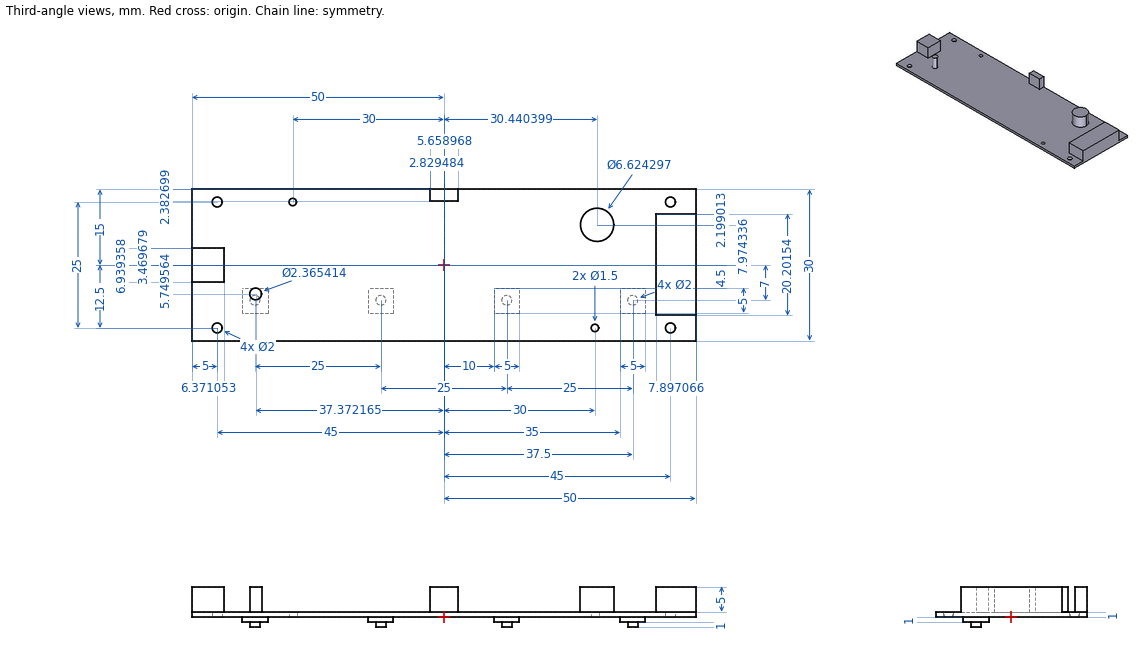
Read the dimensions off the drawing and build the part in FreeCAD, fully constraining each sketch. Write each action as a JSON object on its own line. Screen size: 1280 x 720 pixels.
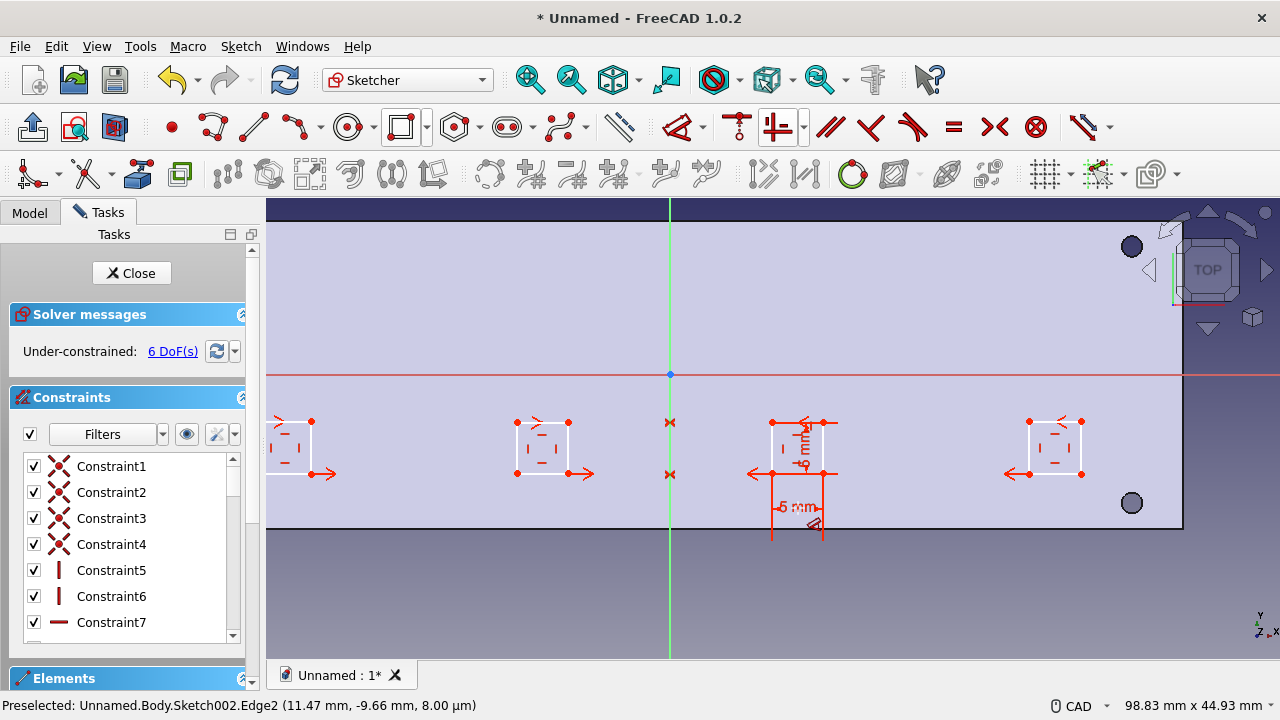
{"action": "left_click", "coordinate": [1029, 437]}
{"action": "left_click", "coordinate": [1063, 448]}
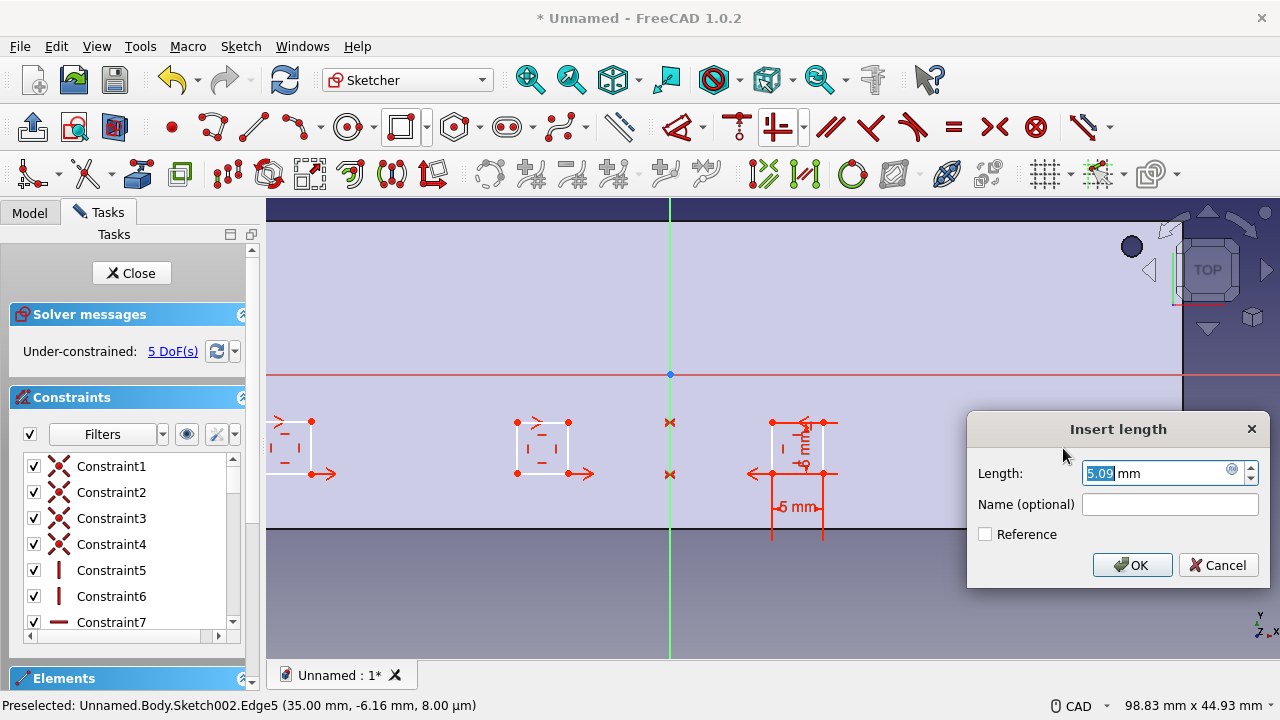
{"action": "type", "text": "5"}
{"action": "key", "text": "Return"}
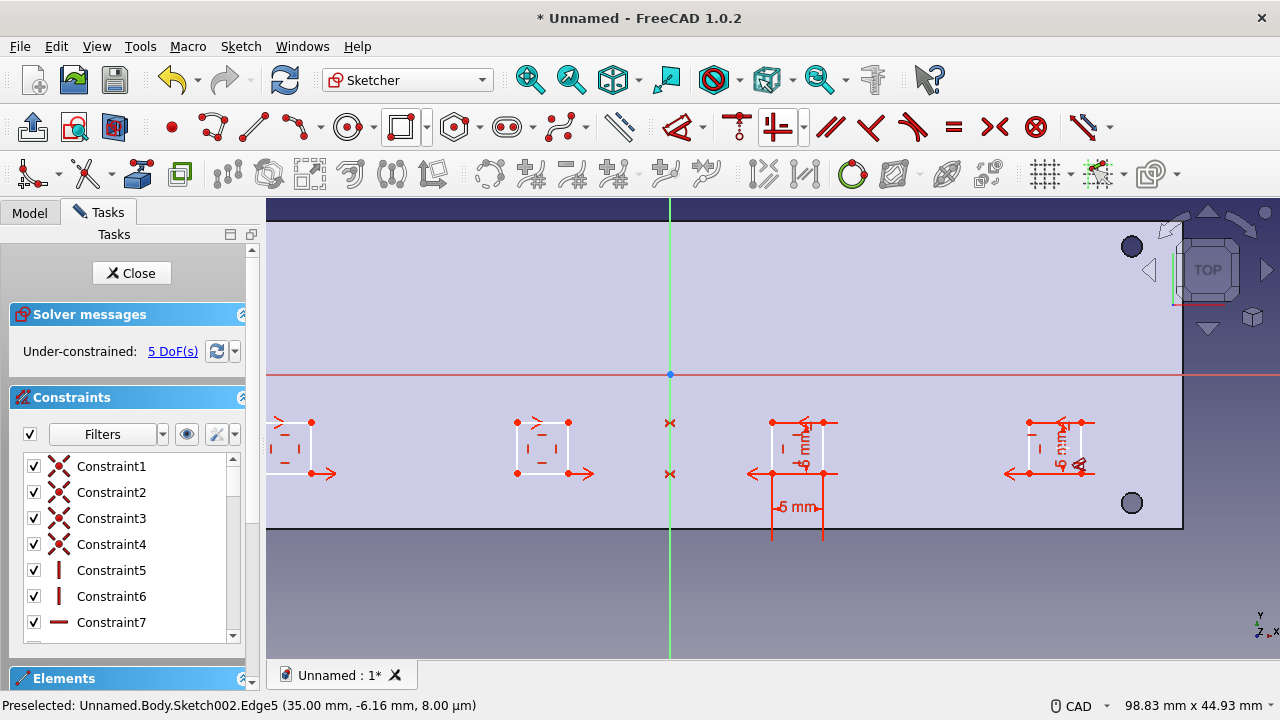
{"action": "left_click", "coordinate": [1045, 474]}
{"action": "left_click", "coordinate": [1055, 508]}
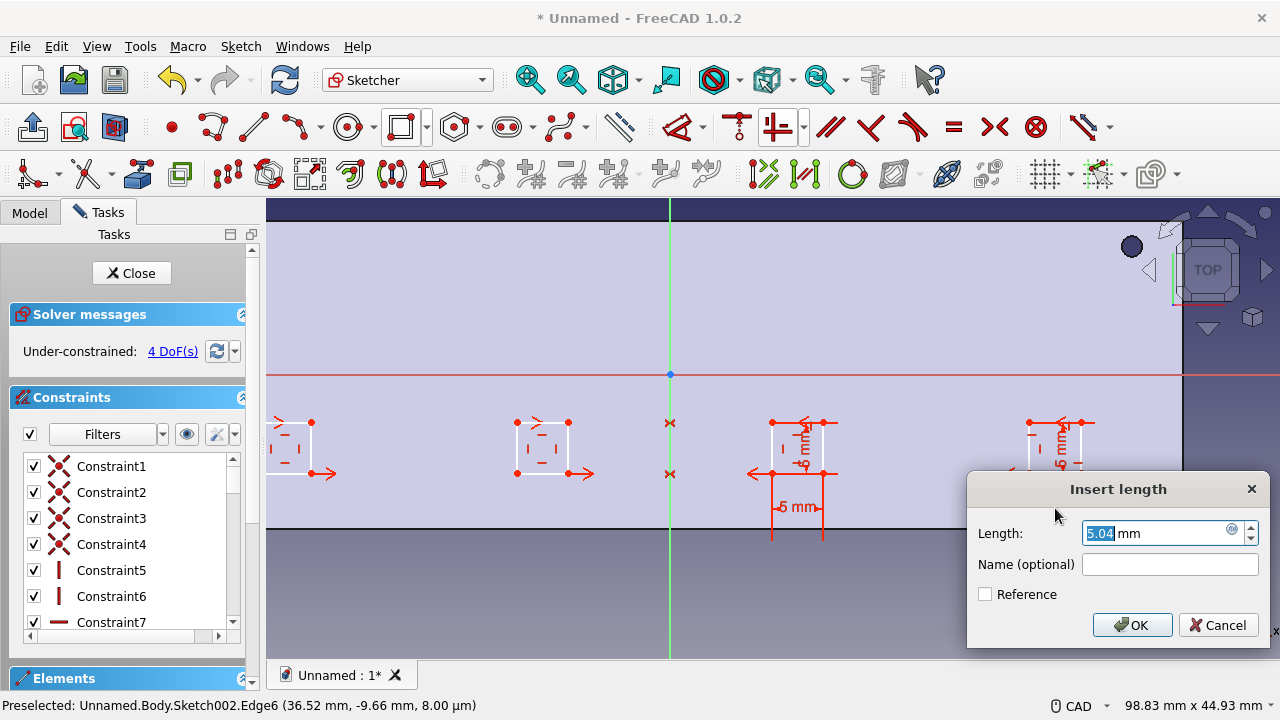
{"action": "type", "text": "5"}
{"action": "key", "text": "Return"}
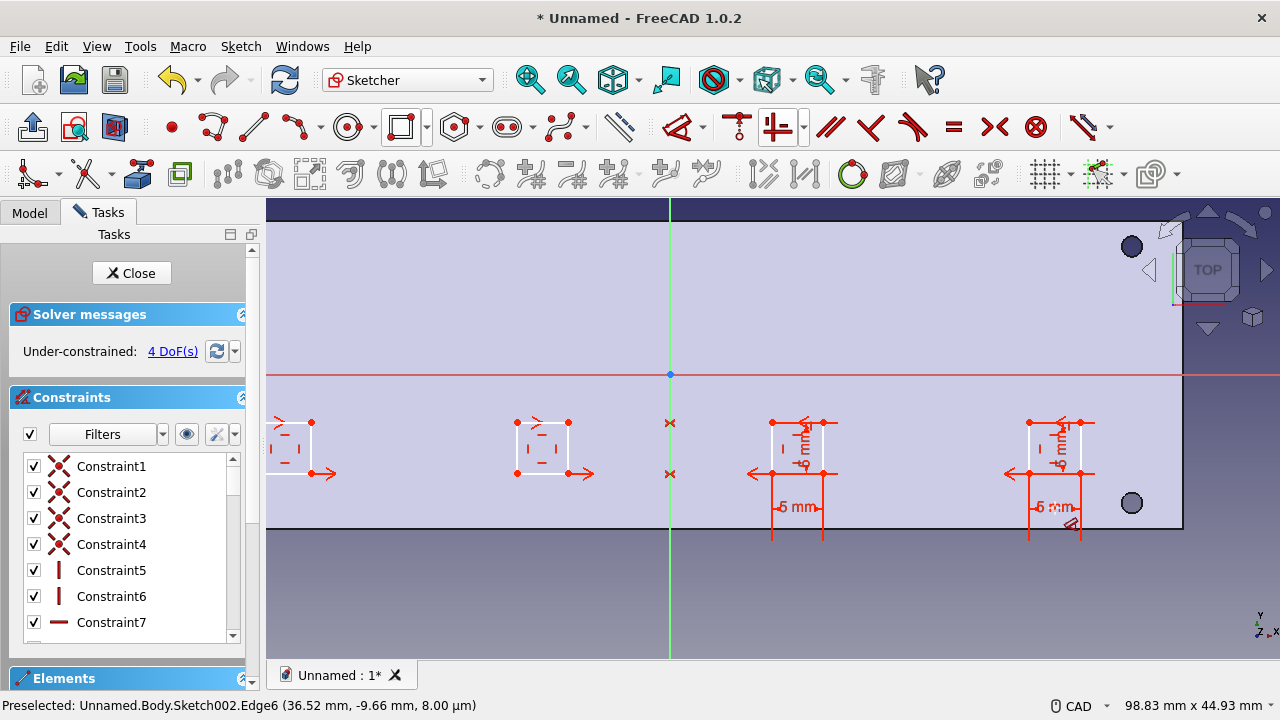
{"action": "left_click", "coordinate": [772, 423]}
{"action": "left_click", "coordinate": [721, 341]}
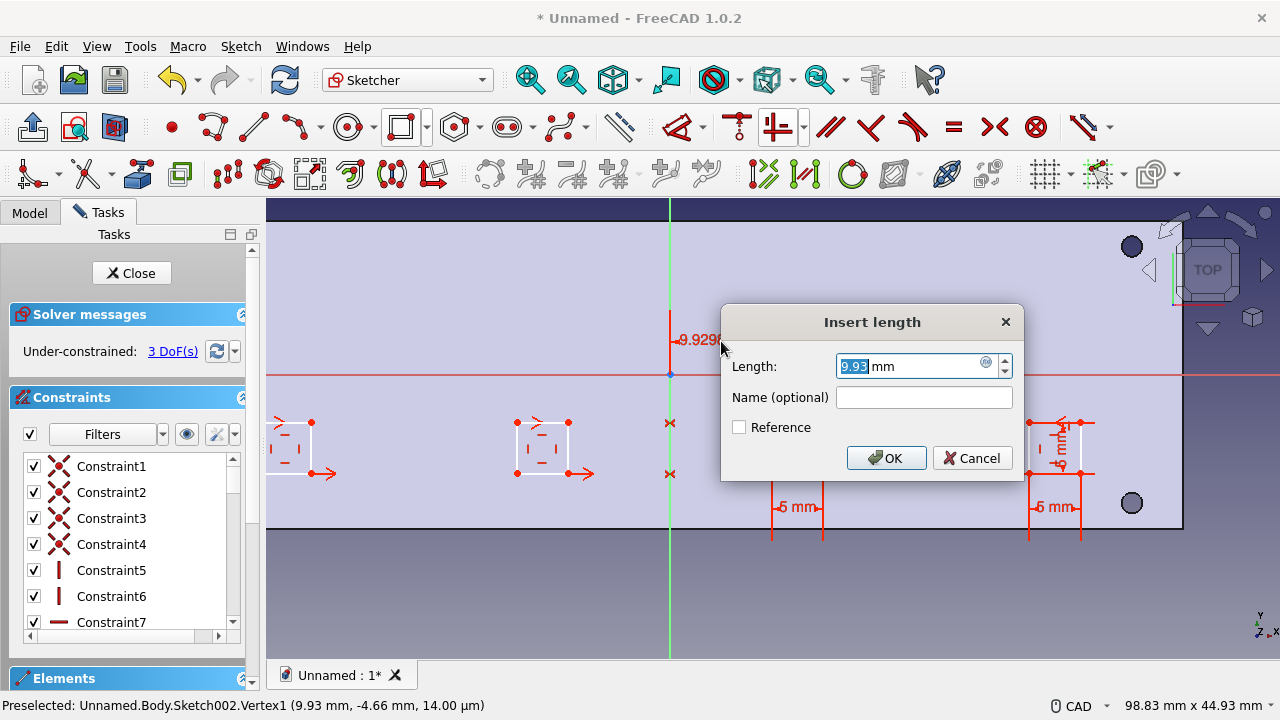
{"action": "type", "text": "10"}
{"action": "key", "text": "Return"}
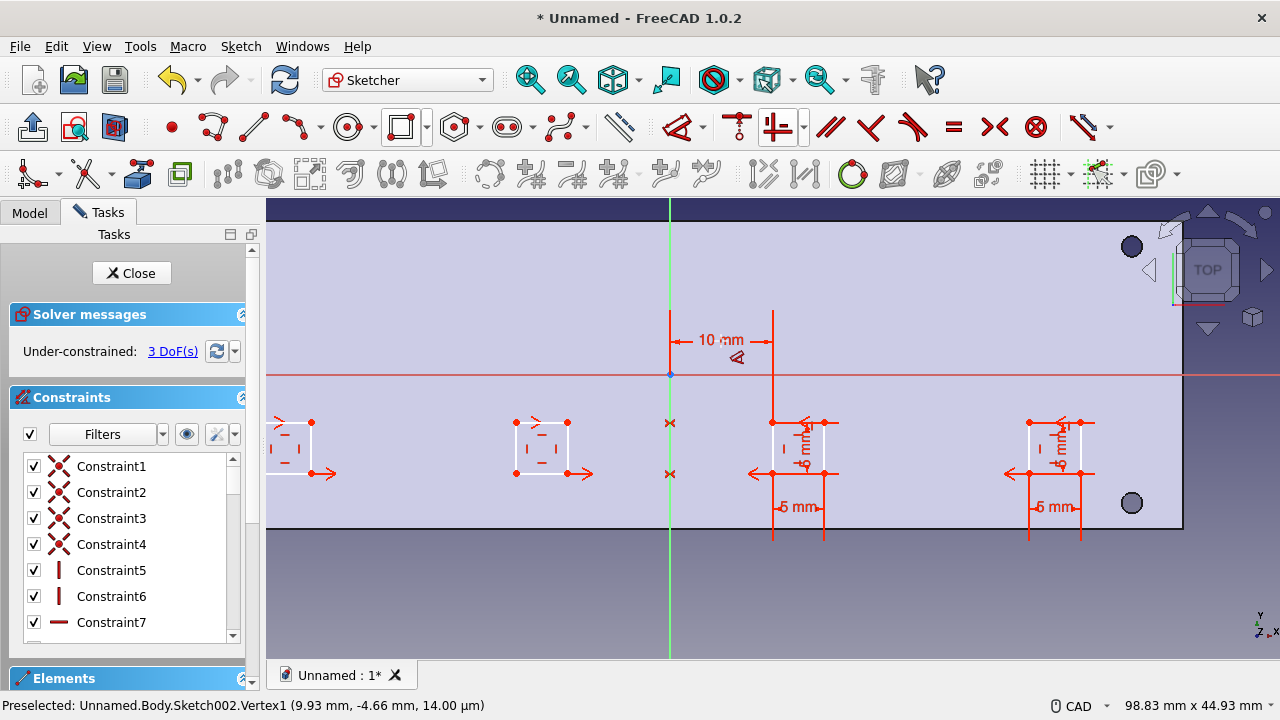
{"action": "left_click", "coordinate": [1029, 423]}
{"action": "left_click", "coordinate": [850, 341]}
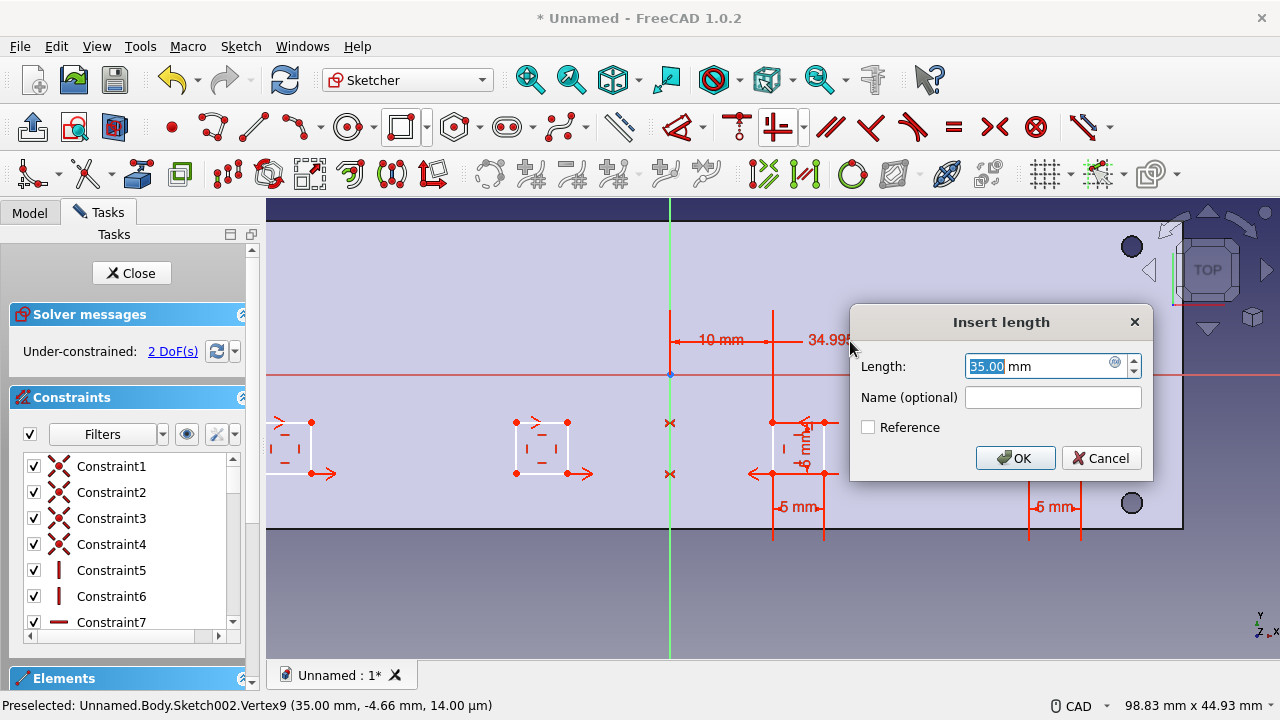
{"action": "type", "text": "35"}
{"action": "key", "text": "Return"}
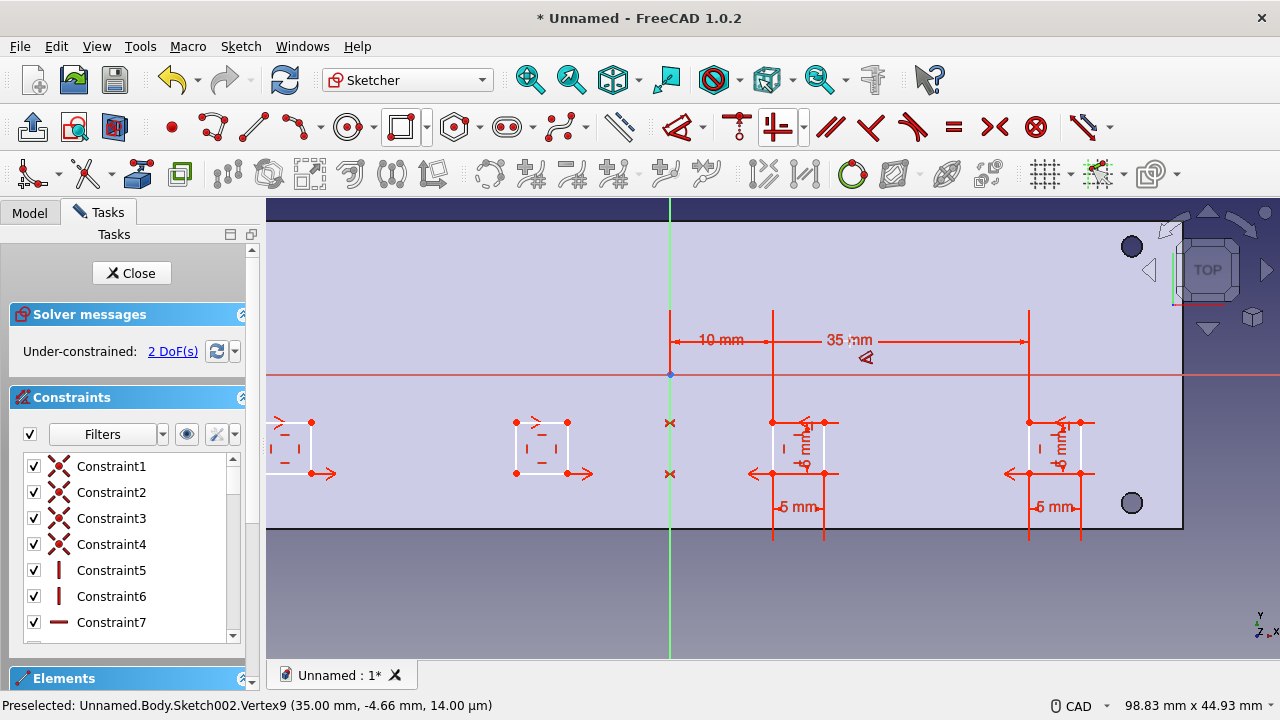
{"action": "left_click", "coordinate": [773, 423]}
{"action": "left_click", "coordinate": [807, 399]}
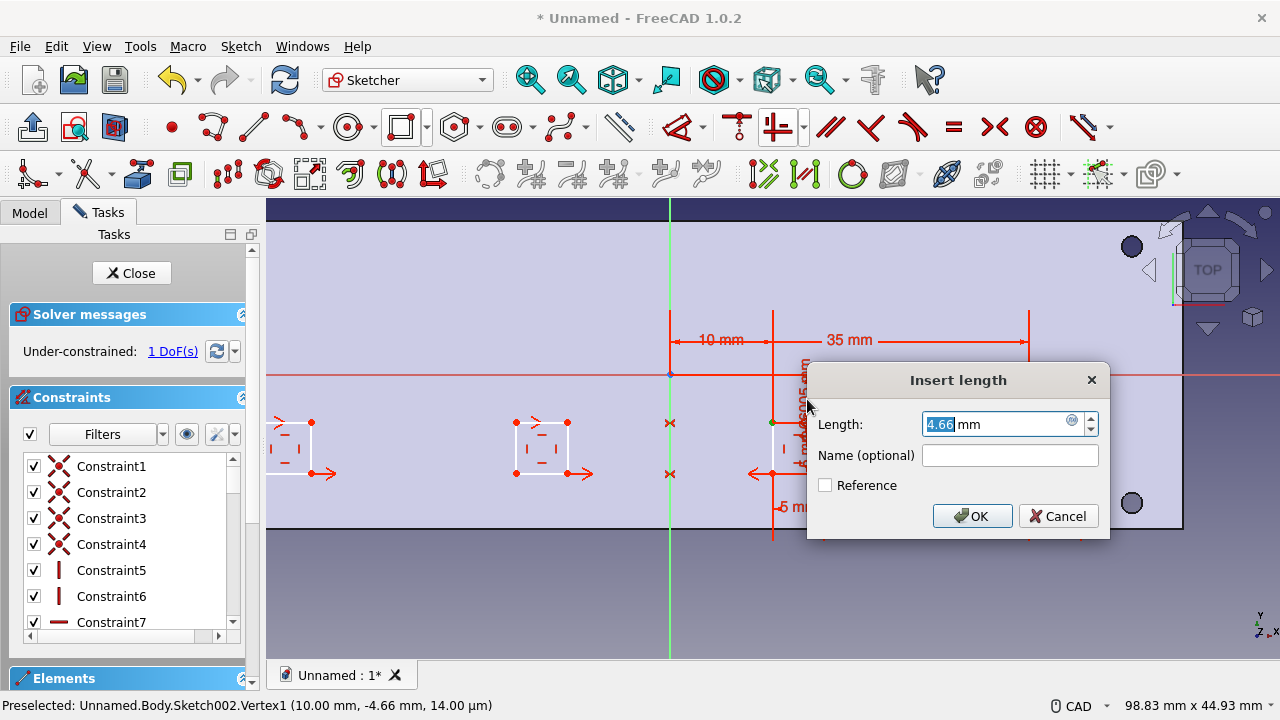
{"action": "type", "text": "4.5"}
{"action": "key", "text": "Return"}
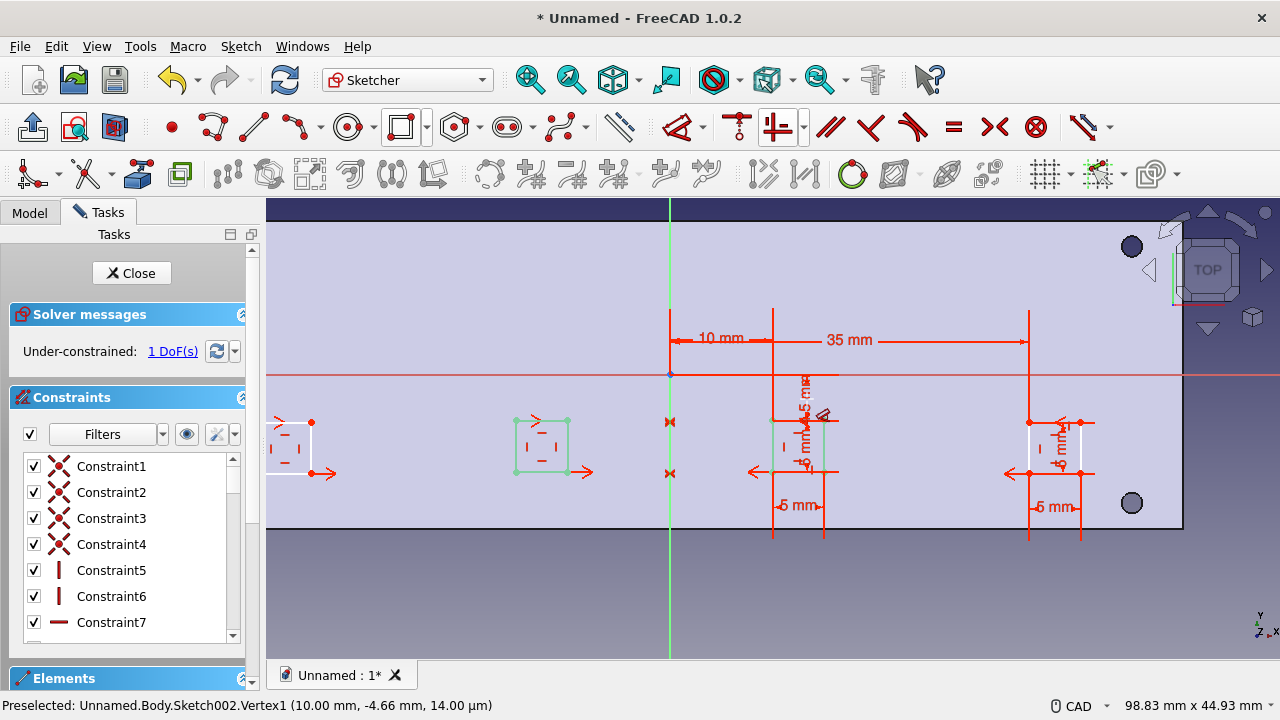
{"action": "left_click", "coordinate": [1029, 423]}
{"action": "left_click", "coordinate": [1063, 399]}